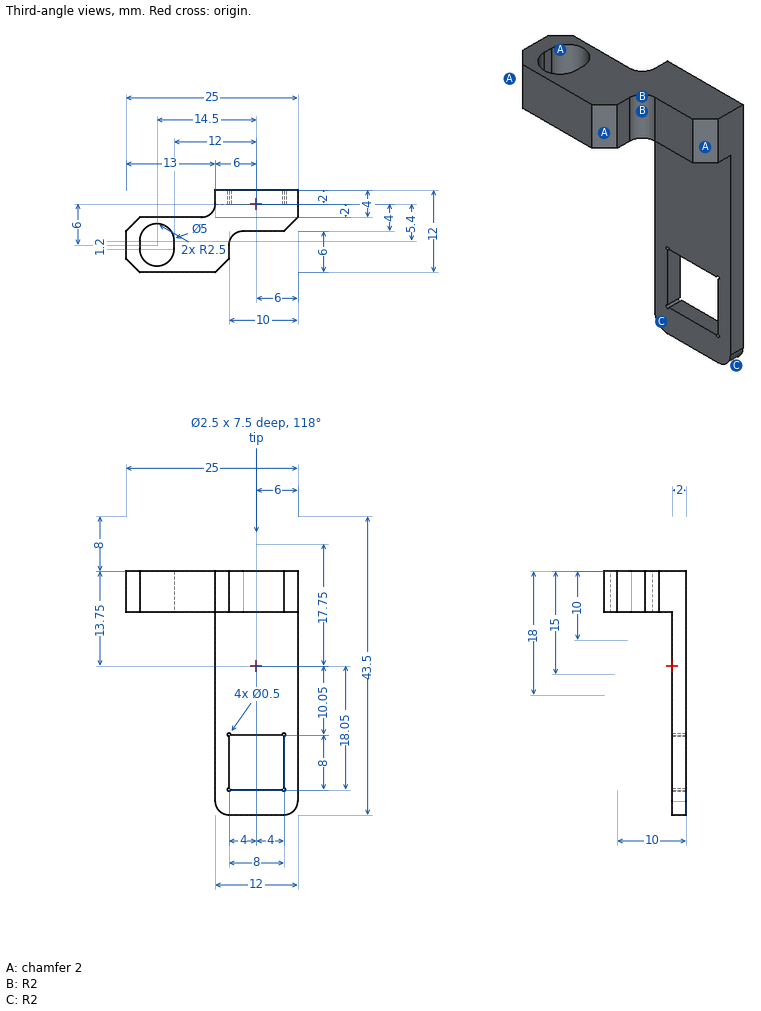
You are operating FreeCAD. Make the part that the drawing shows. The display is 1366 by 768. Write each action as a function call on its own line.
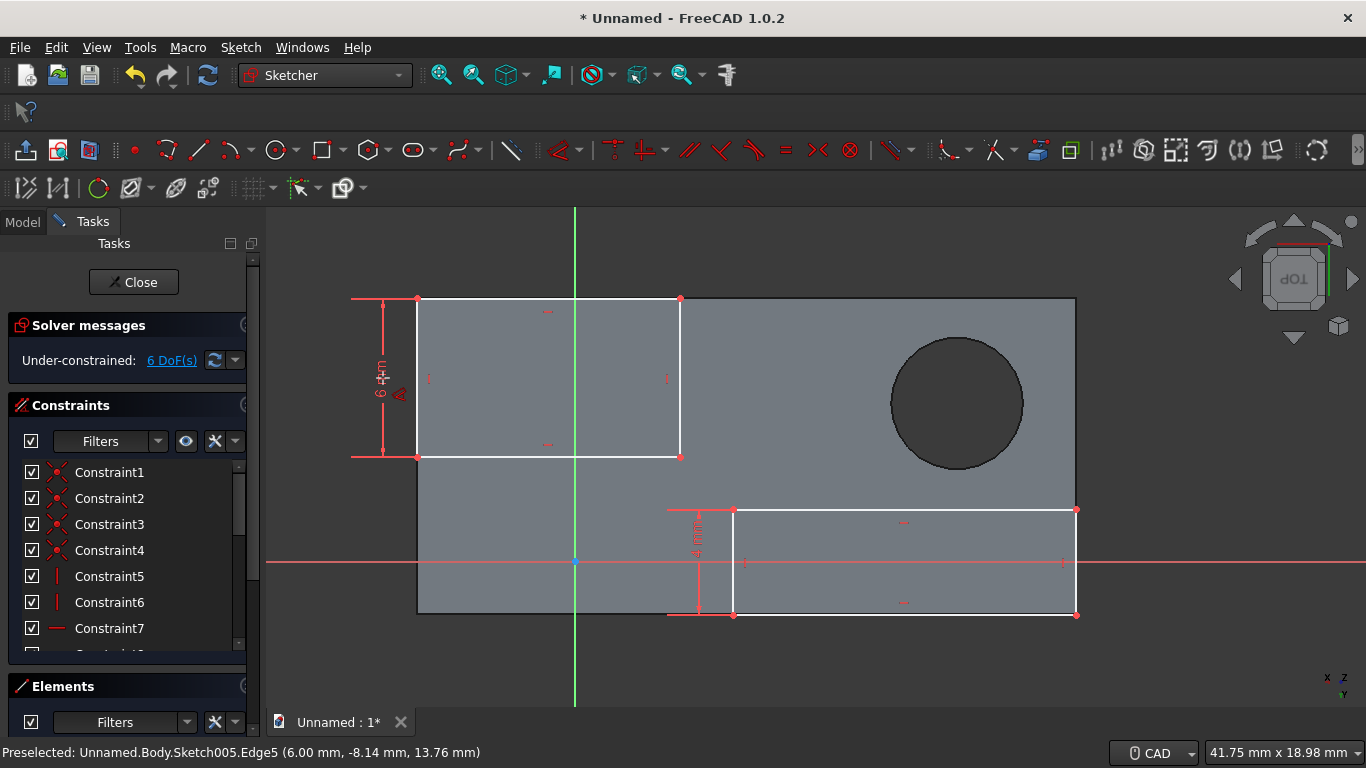
click(836, 615)
click(905, 649)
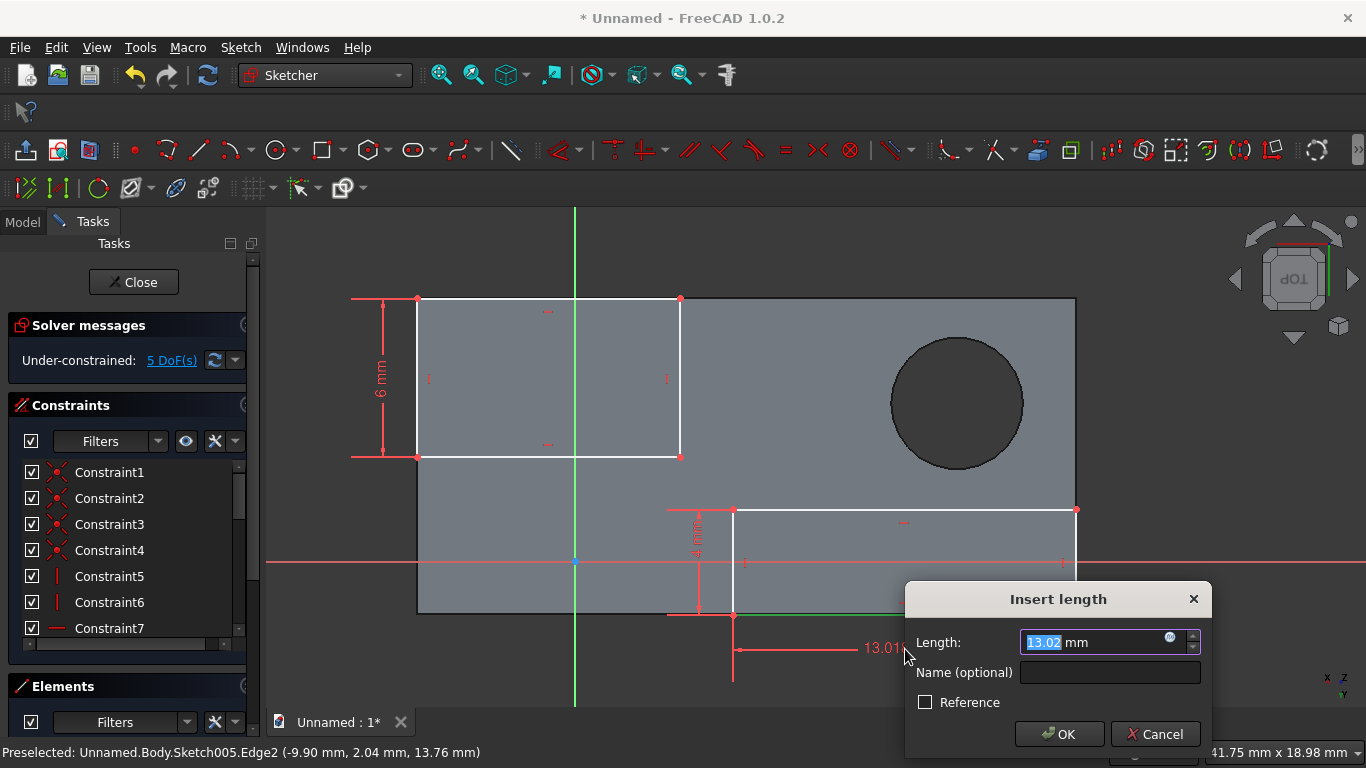
text(13)
key(Return)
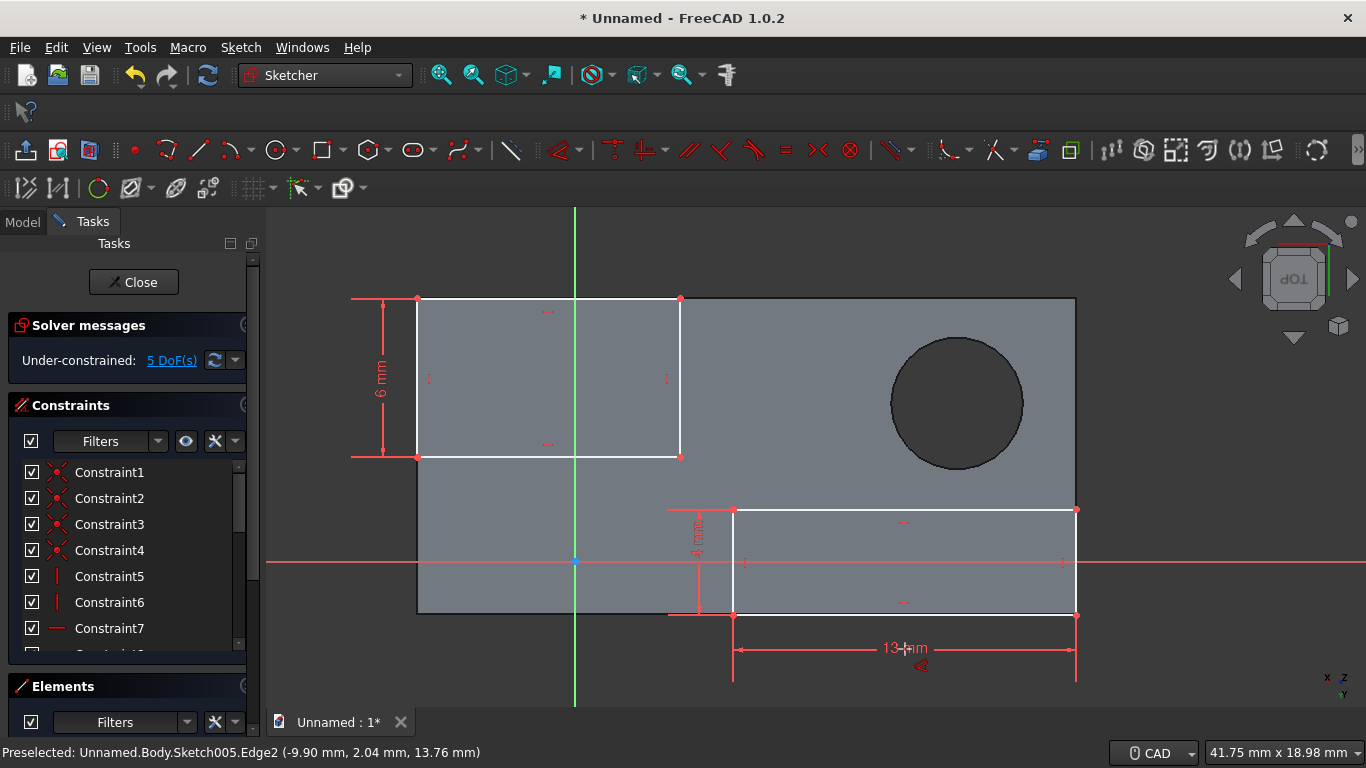
click(496, 457)
click(548, 491)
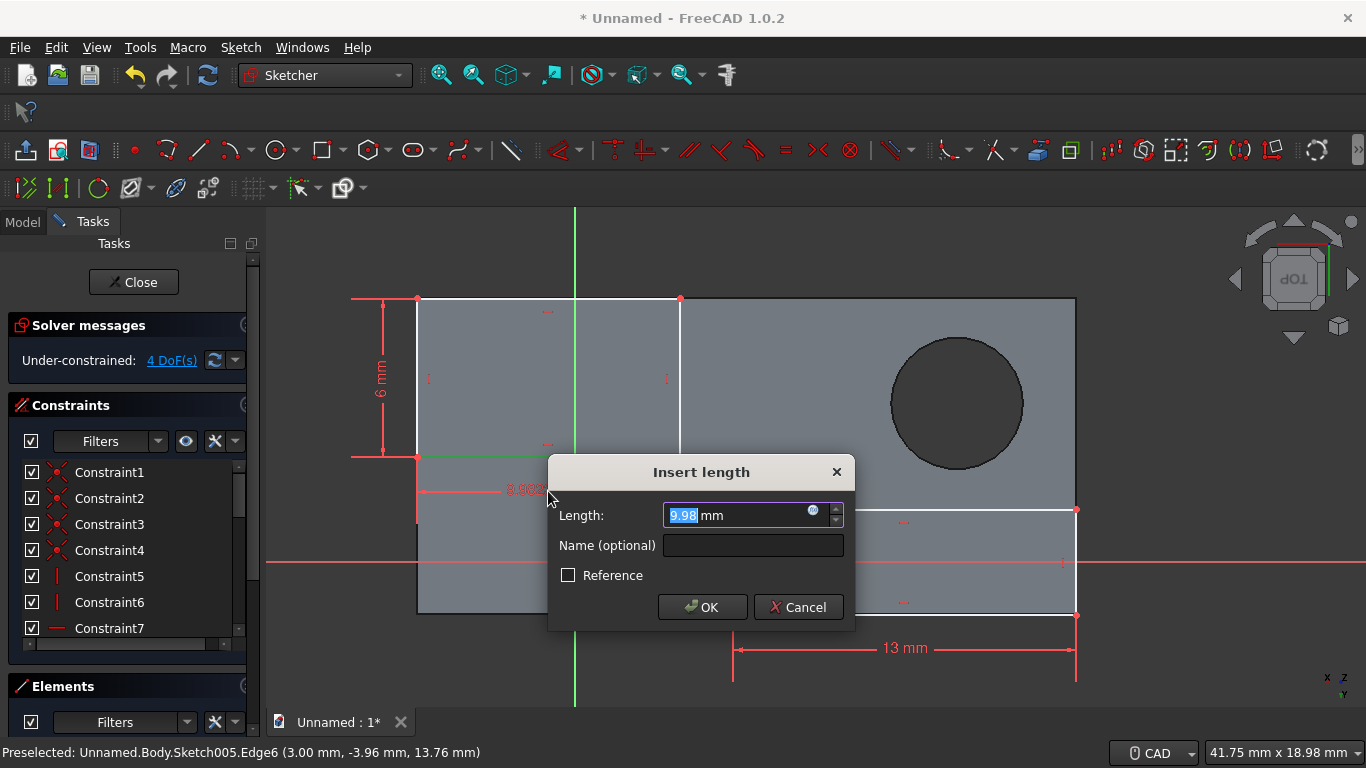
text(10)
key(Return)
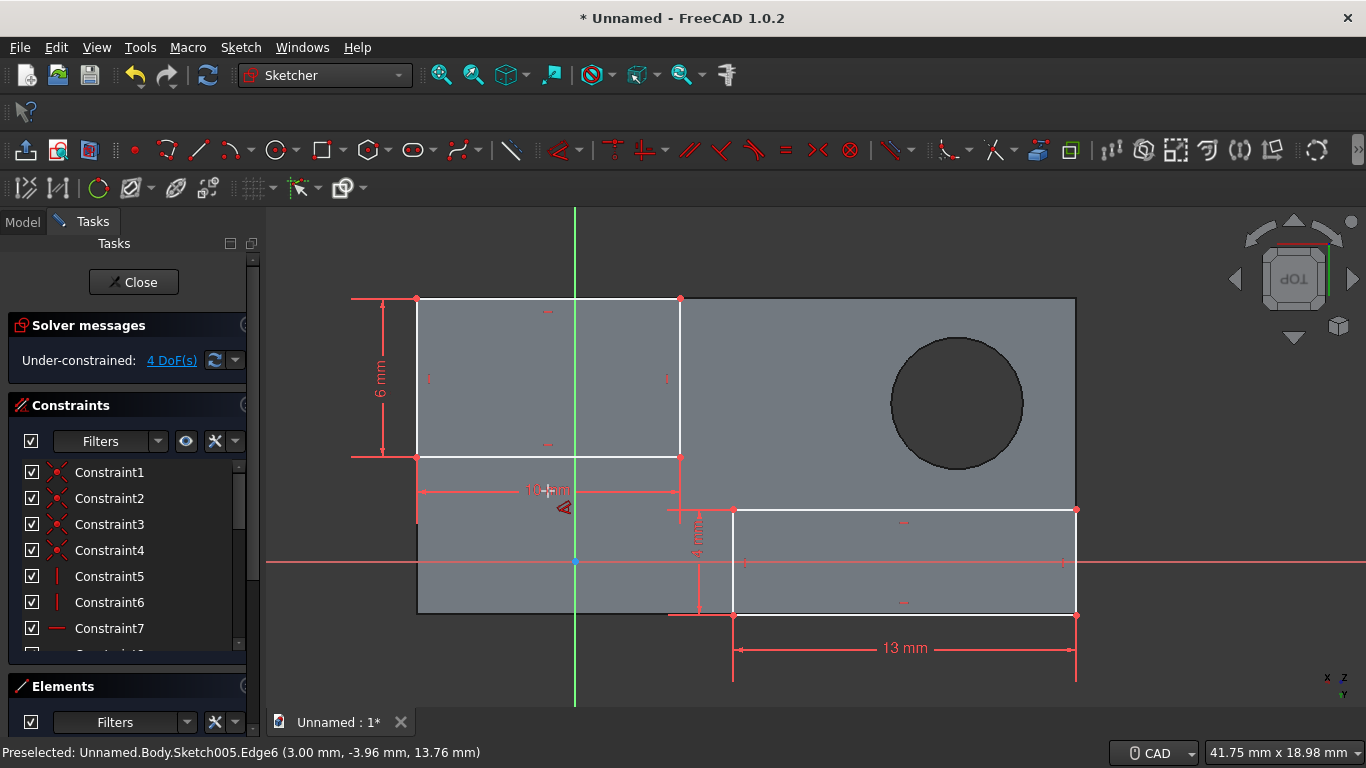
click(733, 510)
click(654, 596)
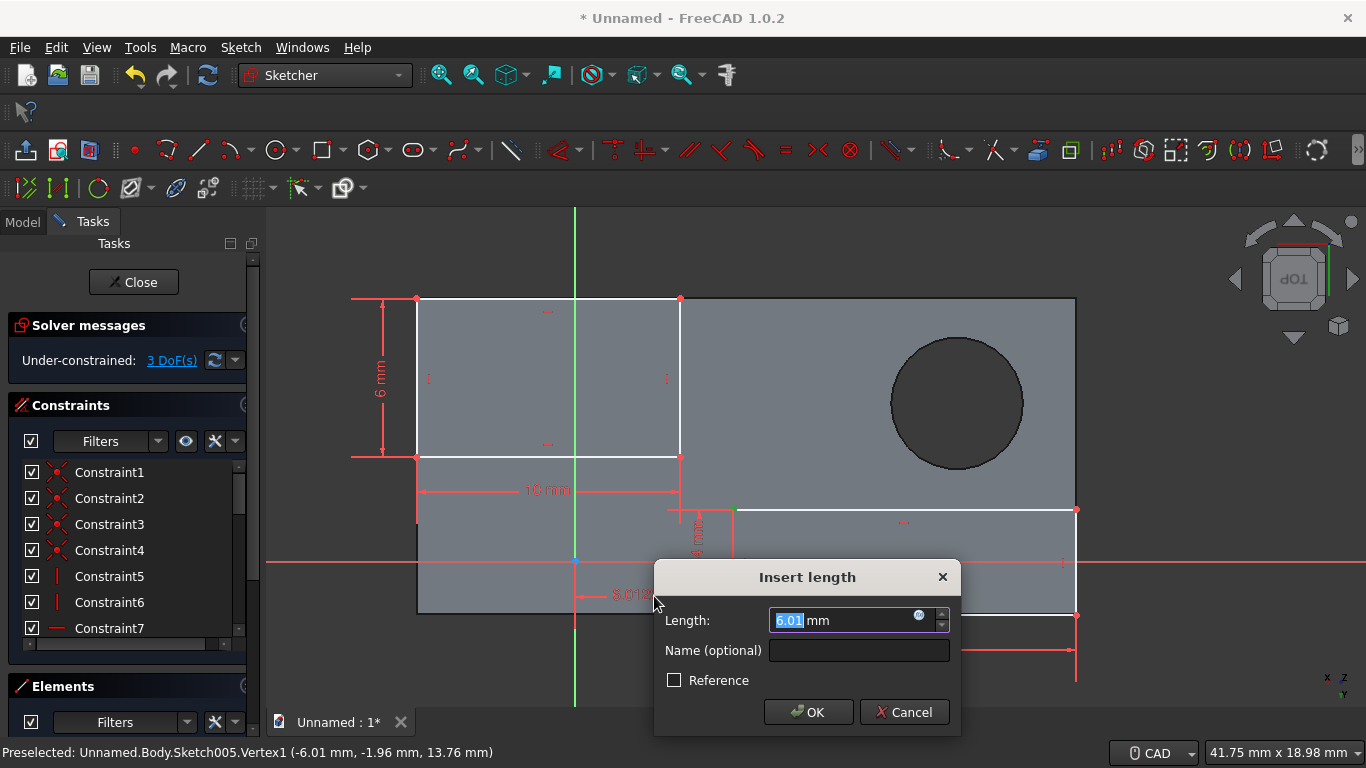
text(6)
key(Return)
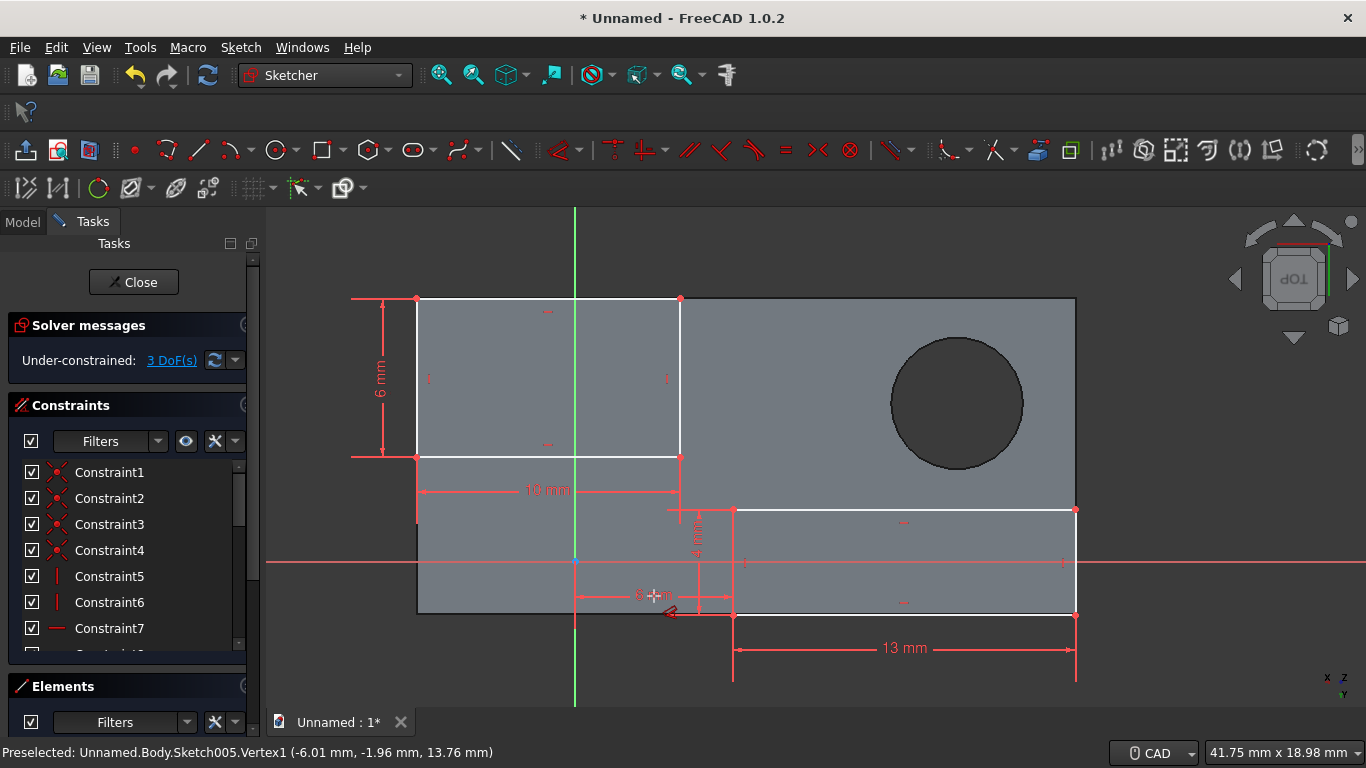
click(733, 510)
click(541, 536)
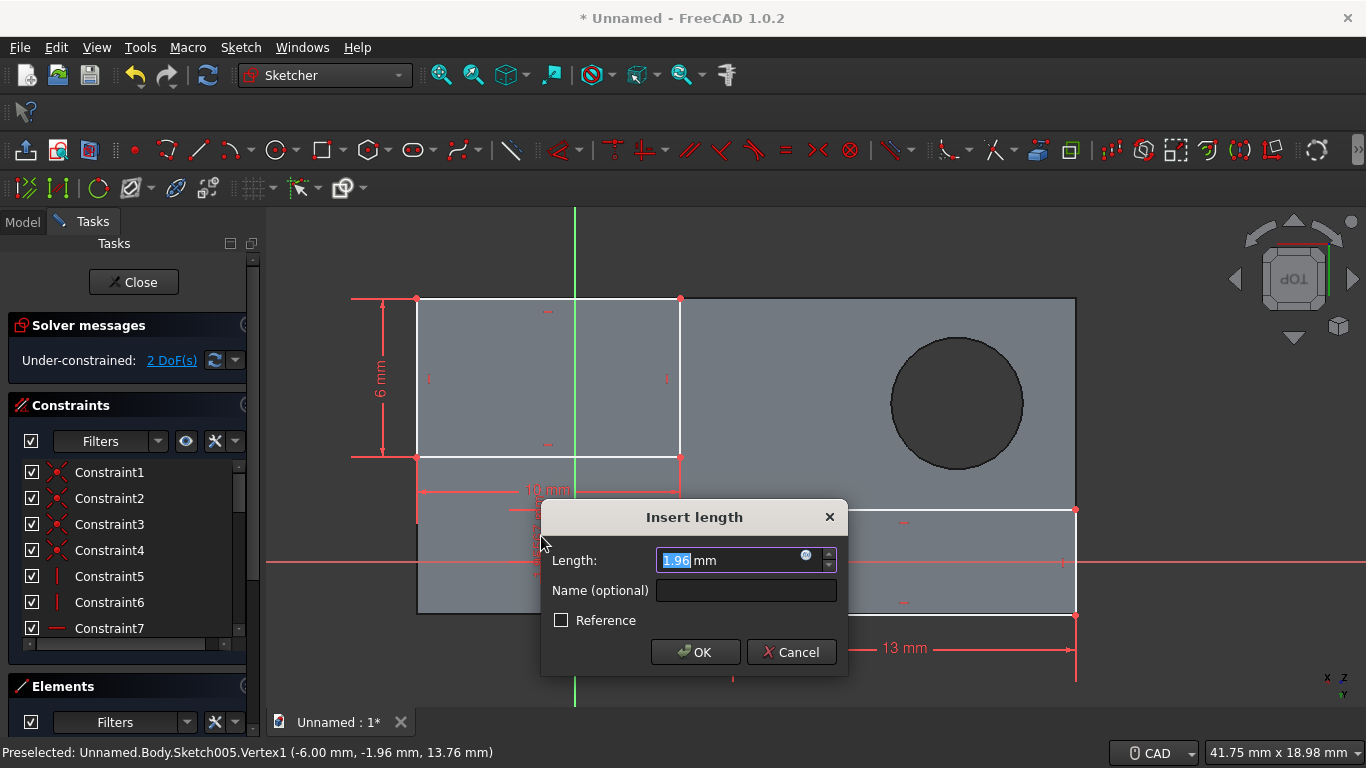
text(2)
key(Return)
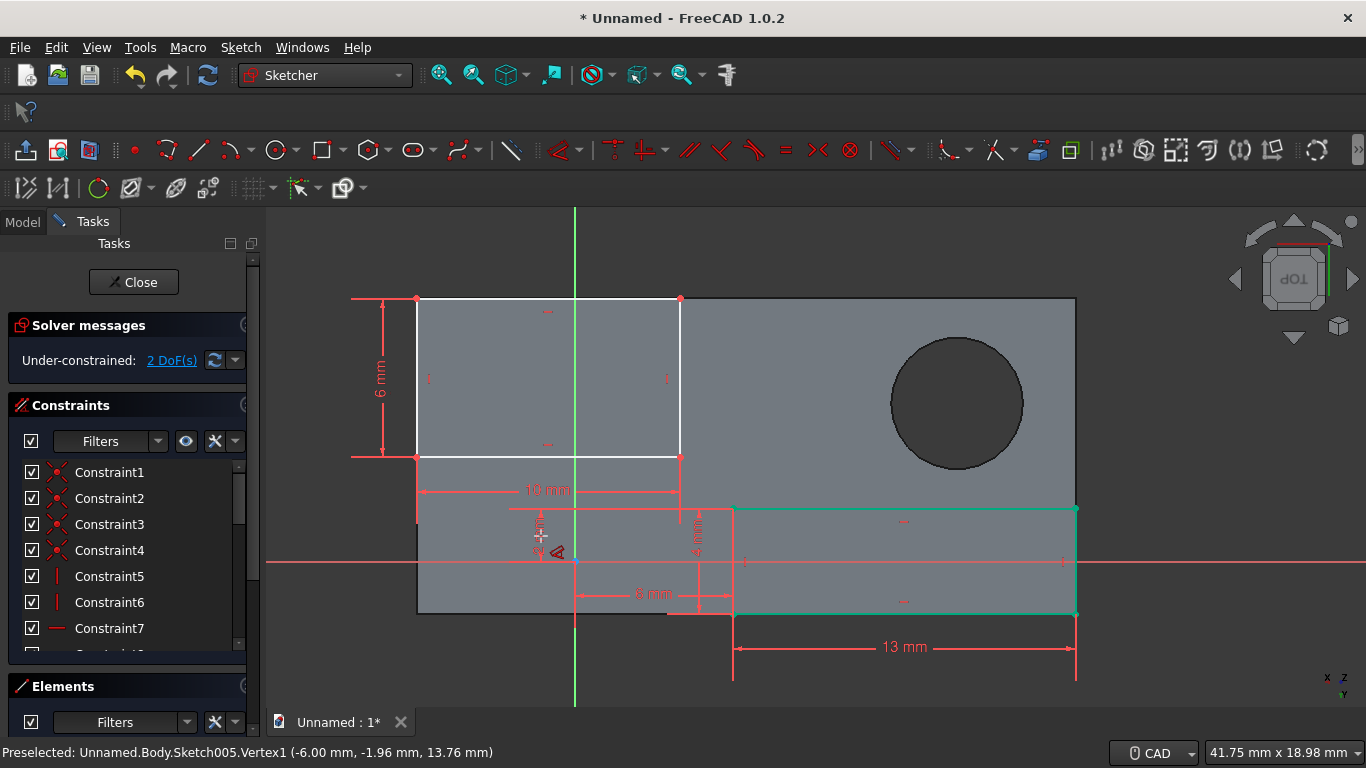
click(417, 299)
click(496, 265)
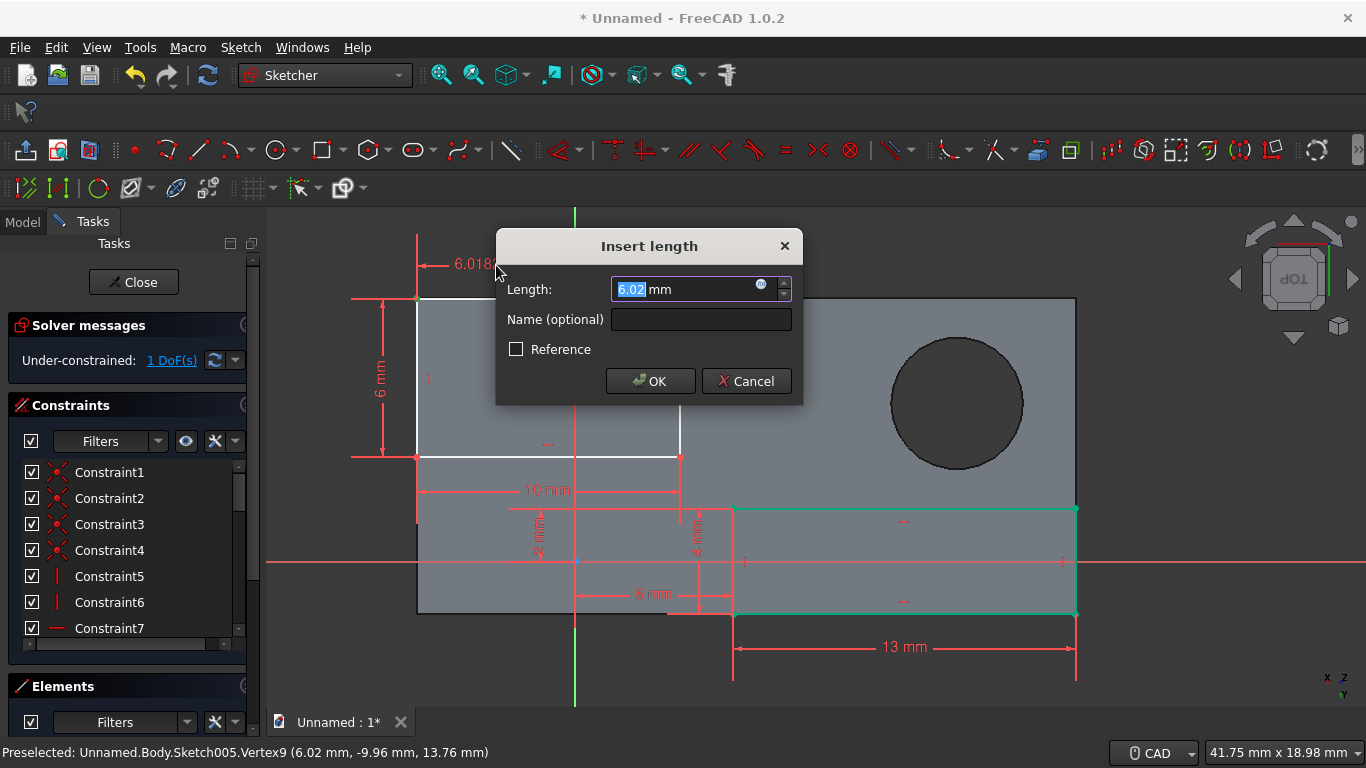
text(6)
key(Return)